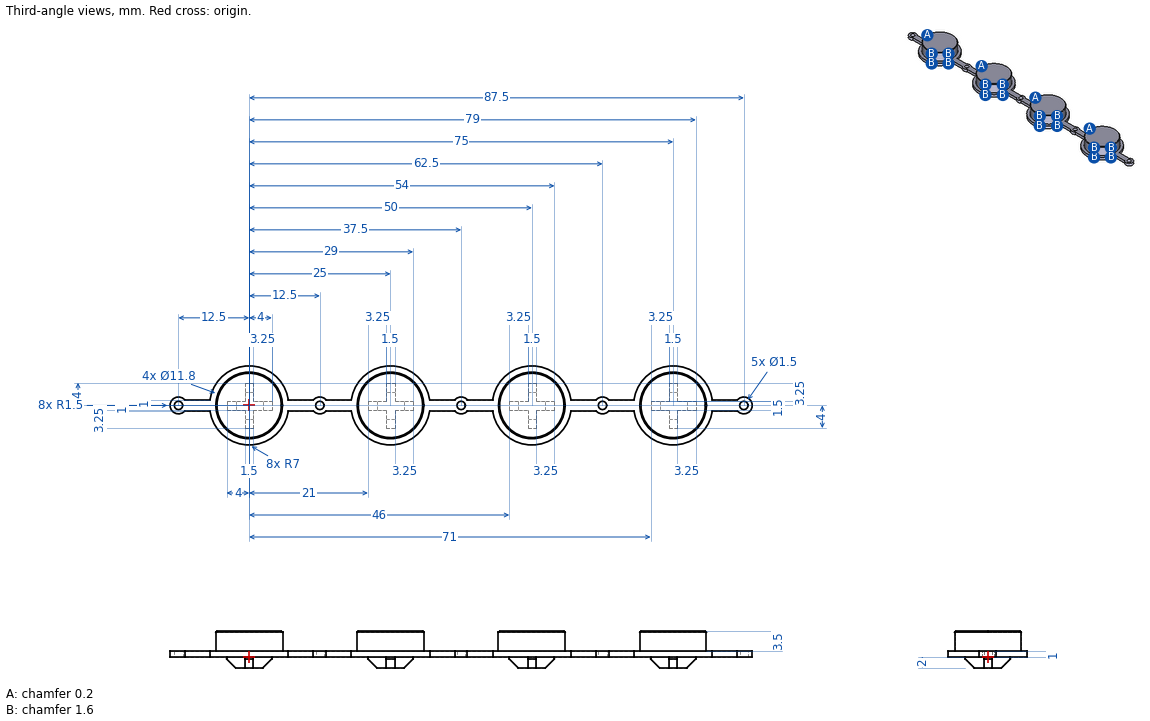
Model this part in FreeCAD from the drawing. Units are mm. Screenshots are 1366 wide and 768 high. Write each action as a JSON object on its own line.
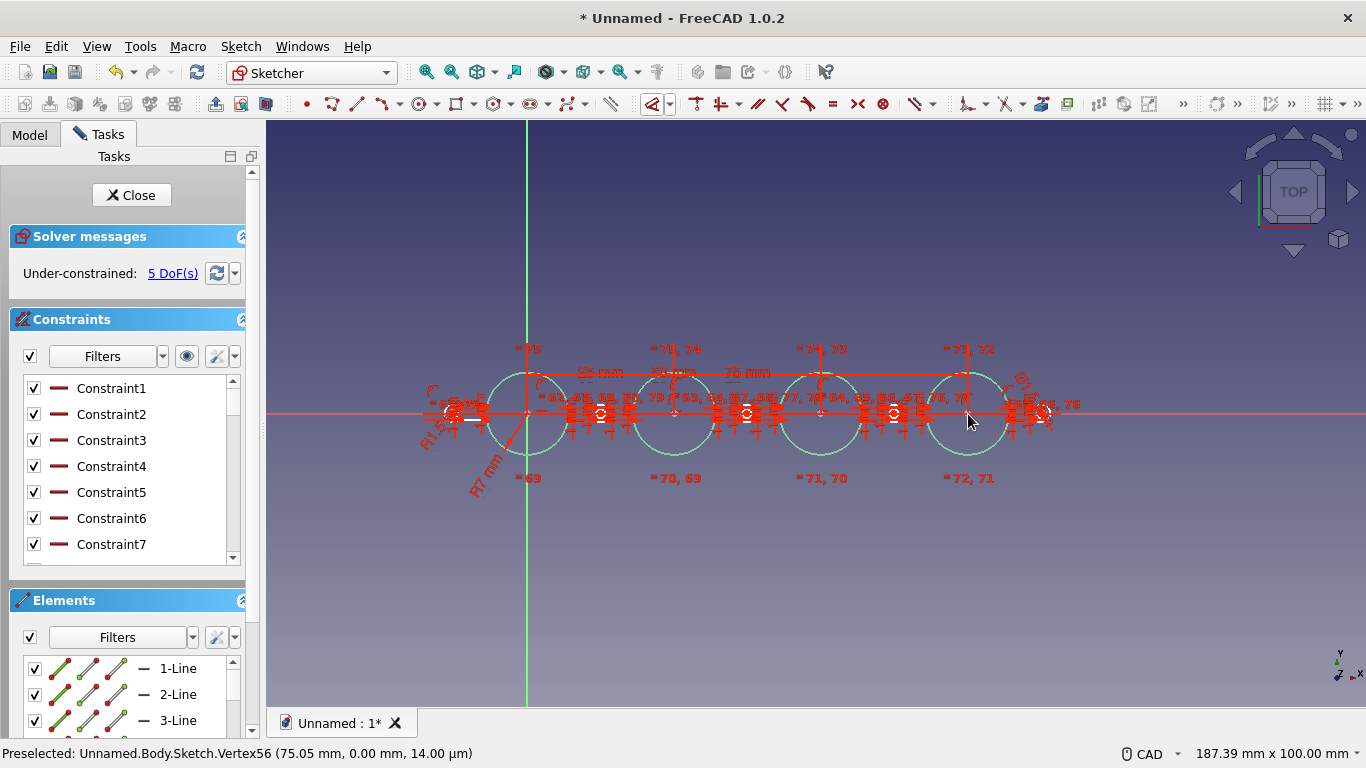
{"action": "scroll", "coordinate": [1041, 414], "scroll_direction": "up", "scroll_amount": 2}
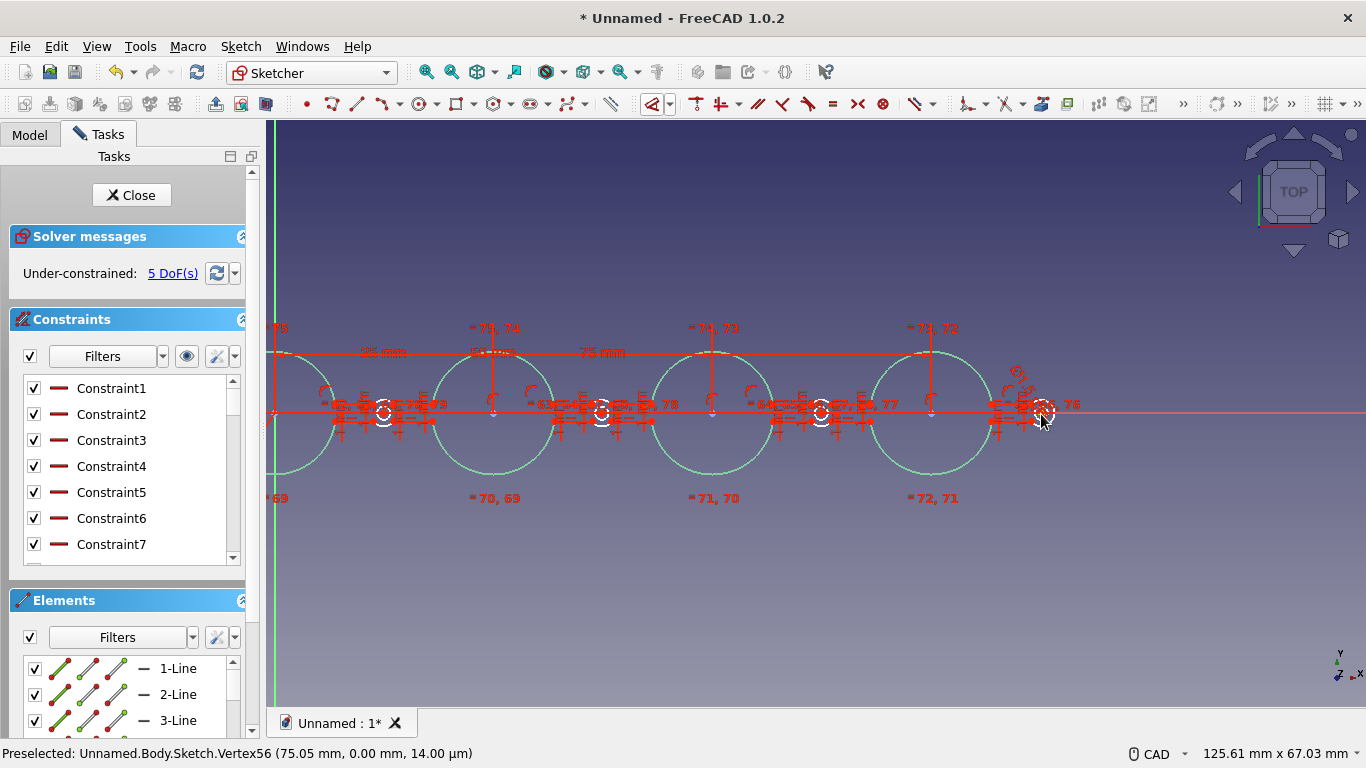
{"action": "left_click", "coordinate": [1041, 413]}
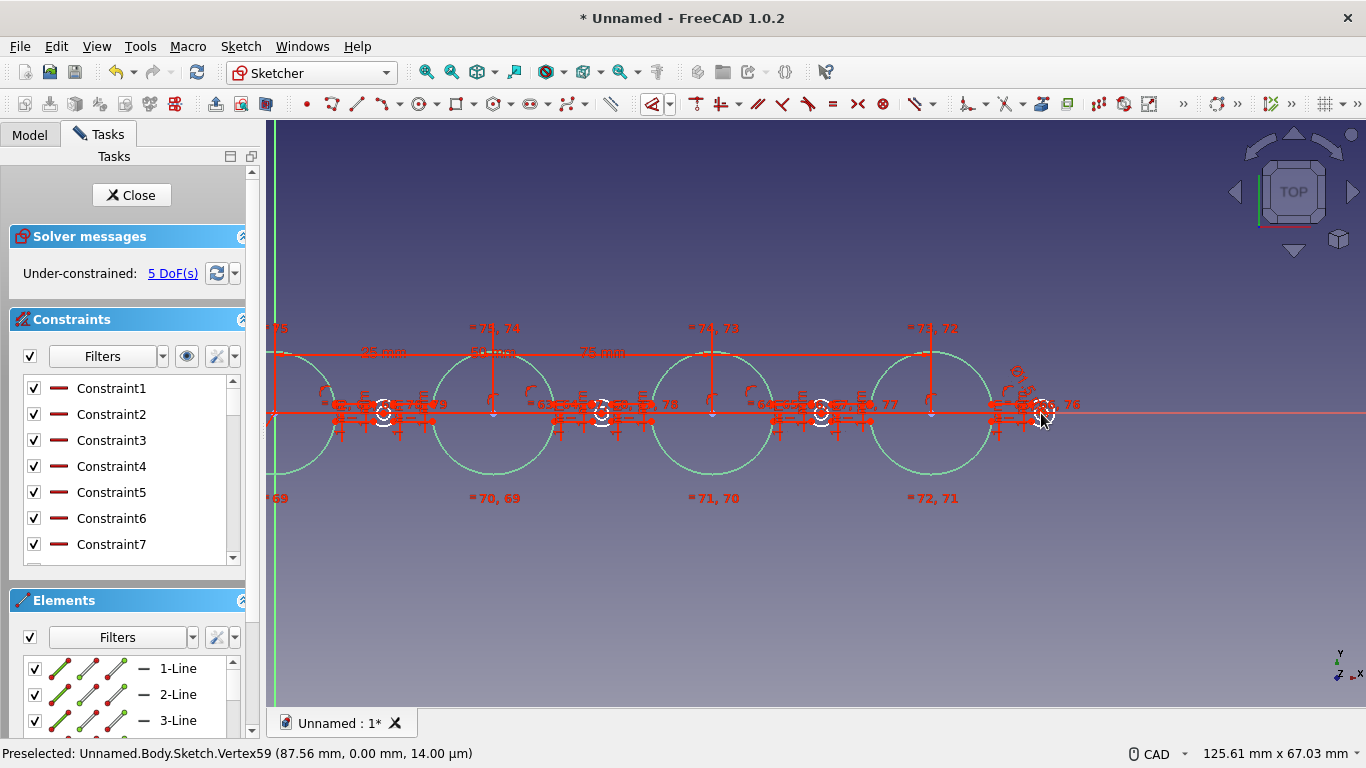
{"action": "key", "text": "l"}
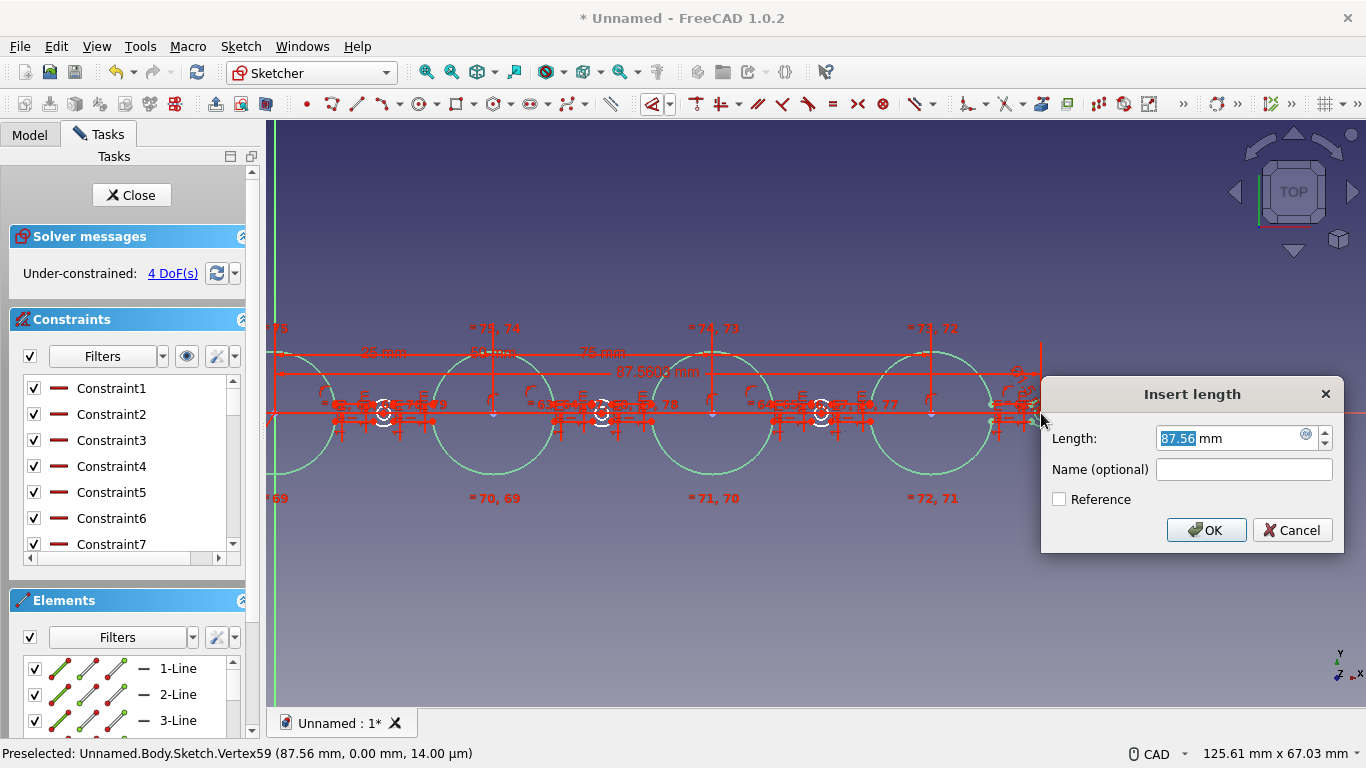
{"action": "type", "text": "87.5"}
{"action": "key", "text": "Return"}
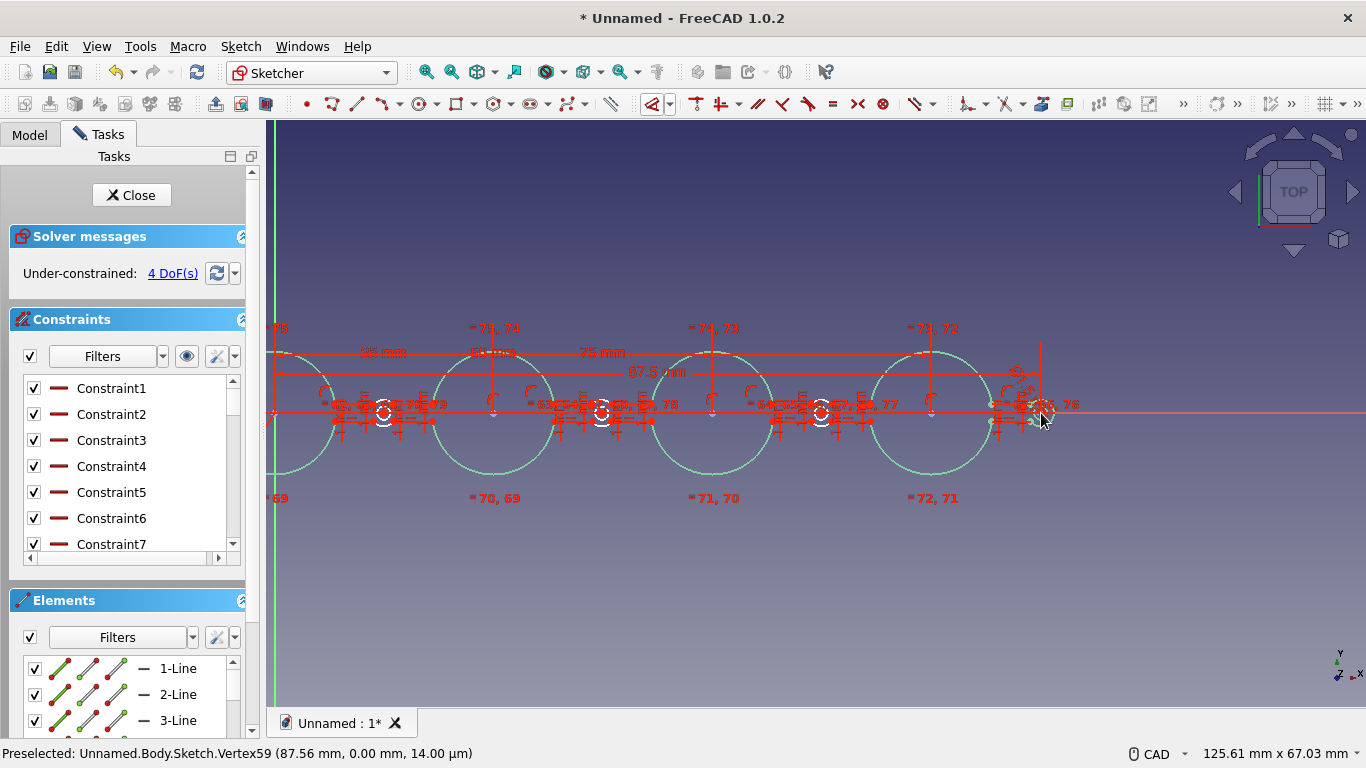
{"action": "left_click", "coordinate": [821, 413]}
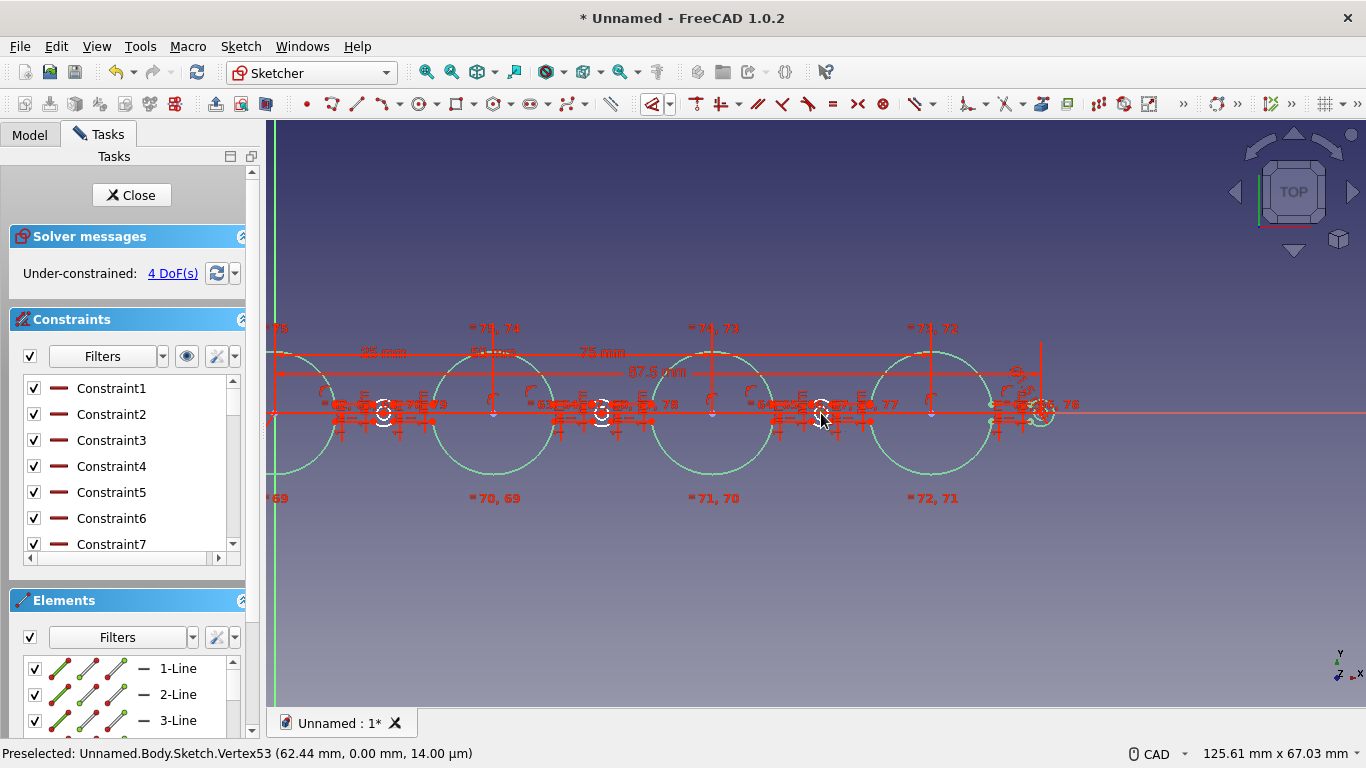
{"action": "key", "text": "l"}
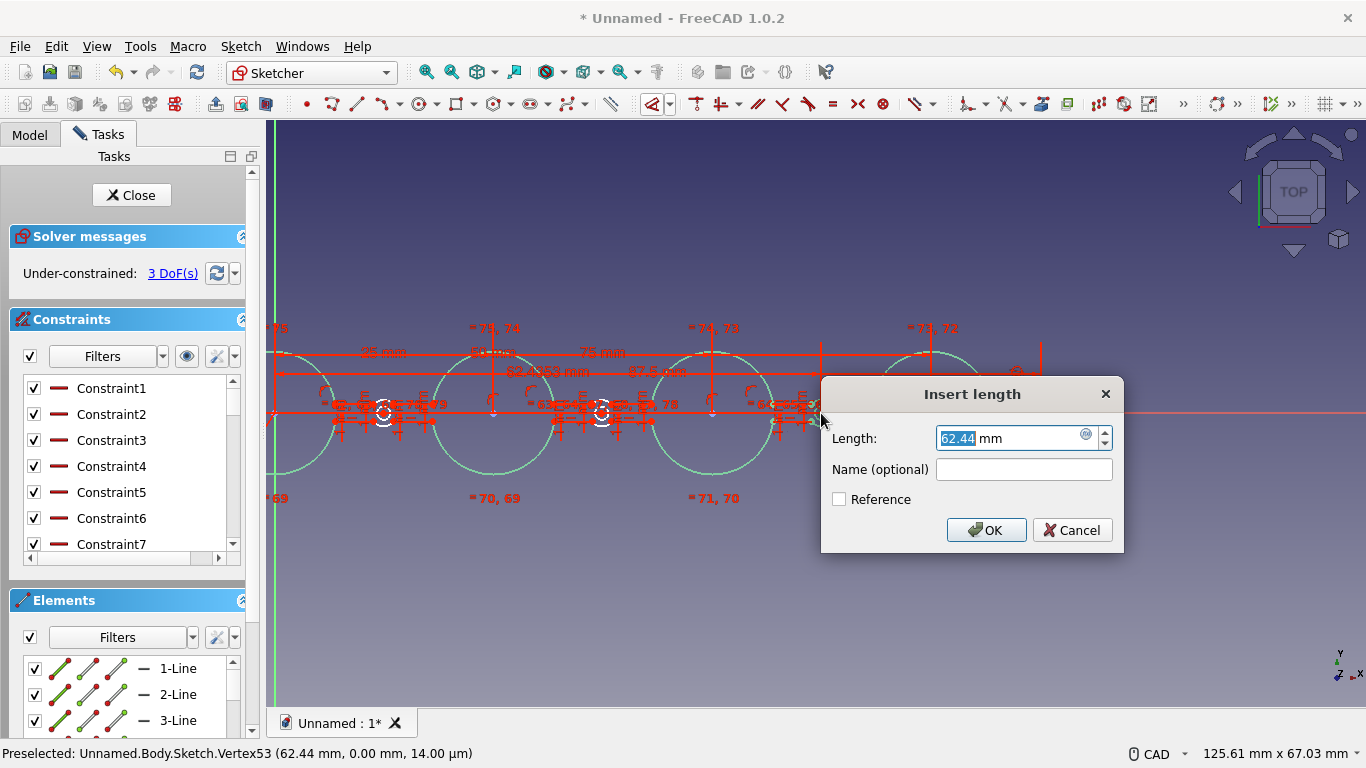
{"action": "type", "text": "62.5"}
{"action": "key", "text": "Return"}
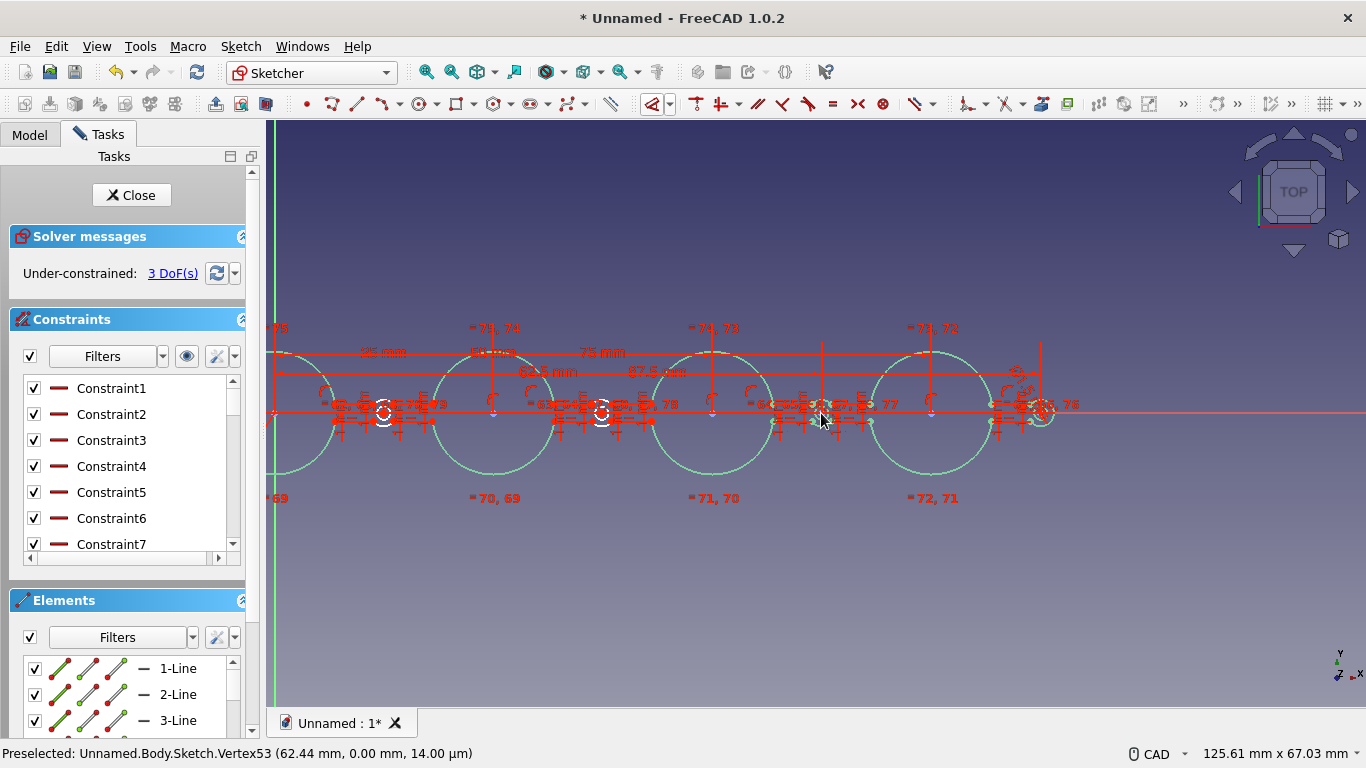
{"action": "left_click", "coordinate": [602, 413]}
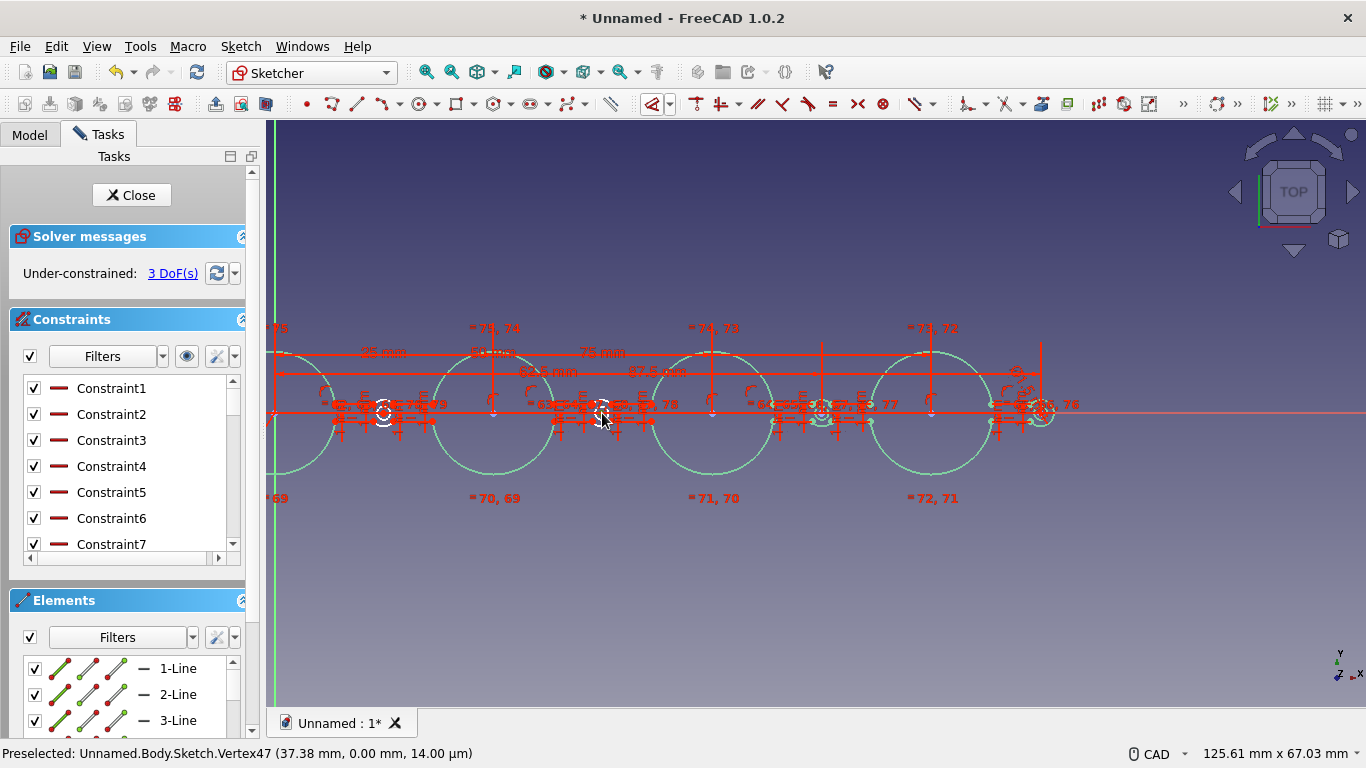
{"action": "key", "text": "l"}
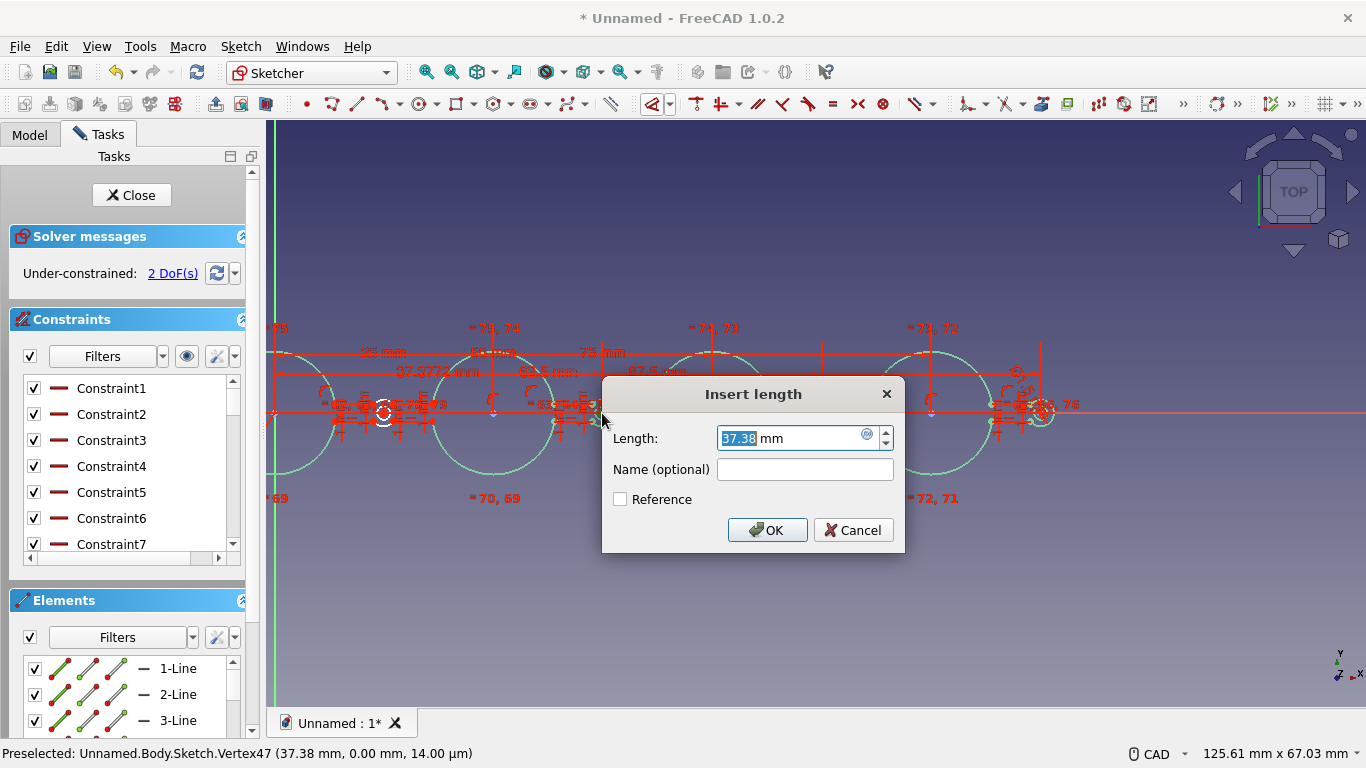
{"action": "type", "text": "37.5"}
{"action": "key", "text": "Return"}